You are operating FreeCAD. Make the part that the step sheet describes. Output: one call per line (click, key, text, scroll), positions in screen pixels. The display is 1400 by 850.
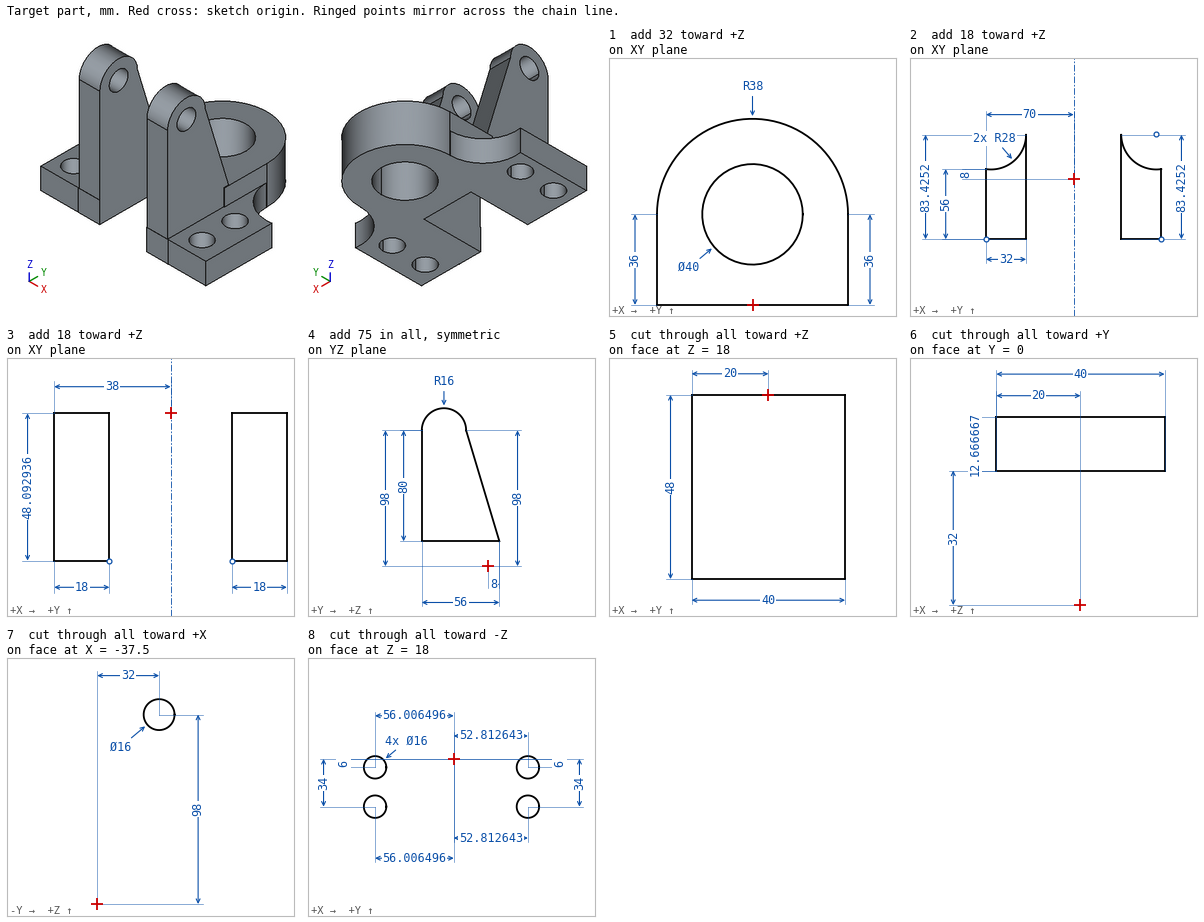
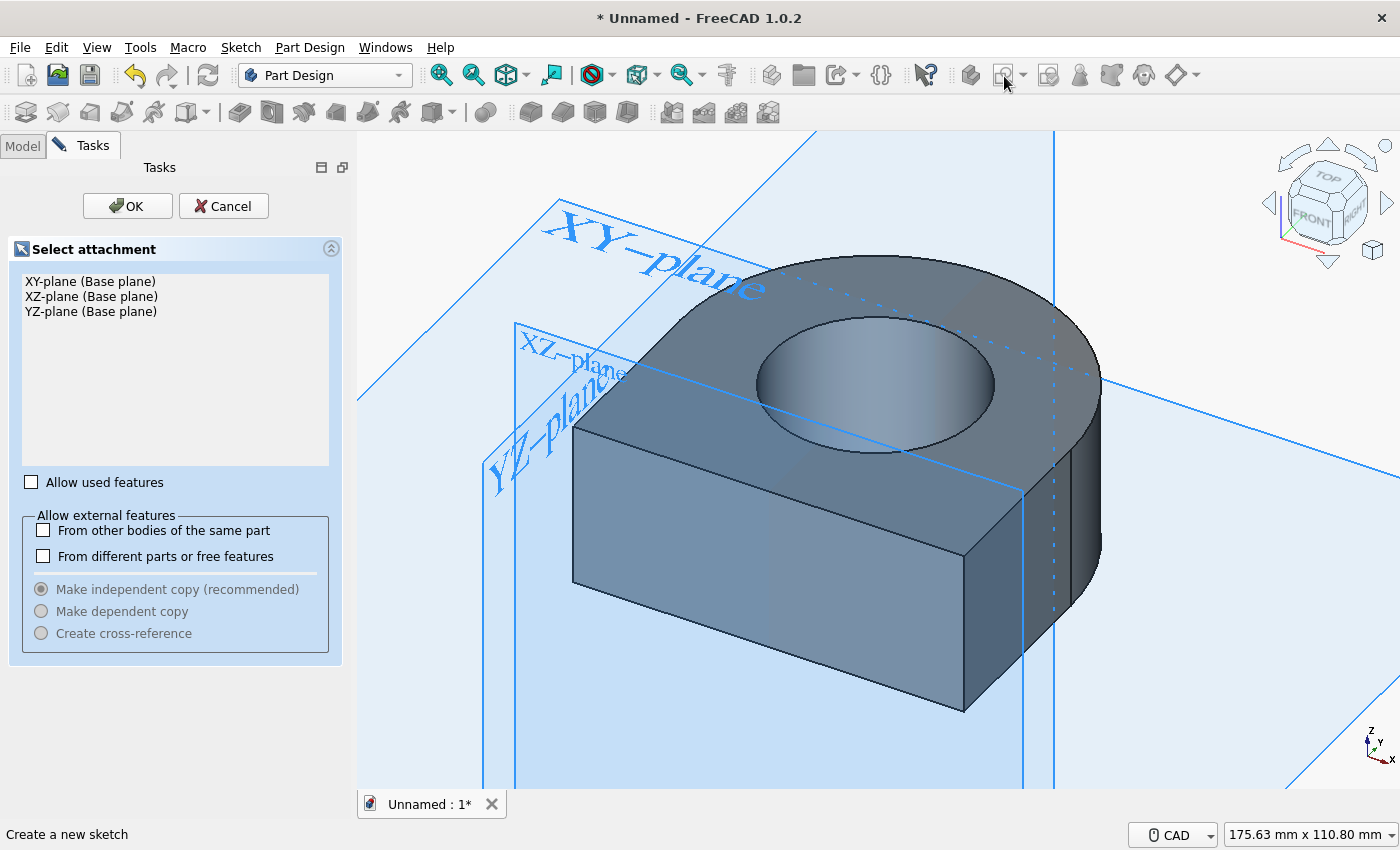
click(82, 282)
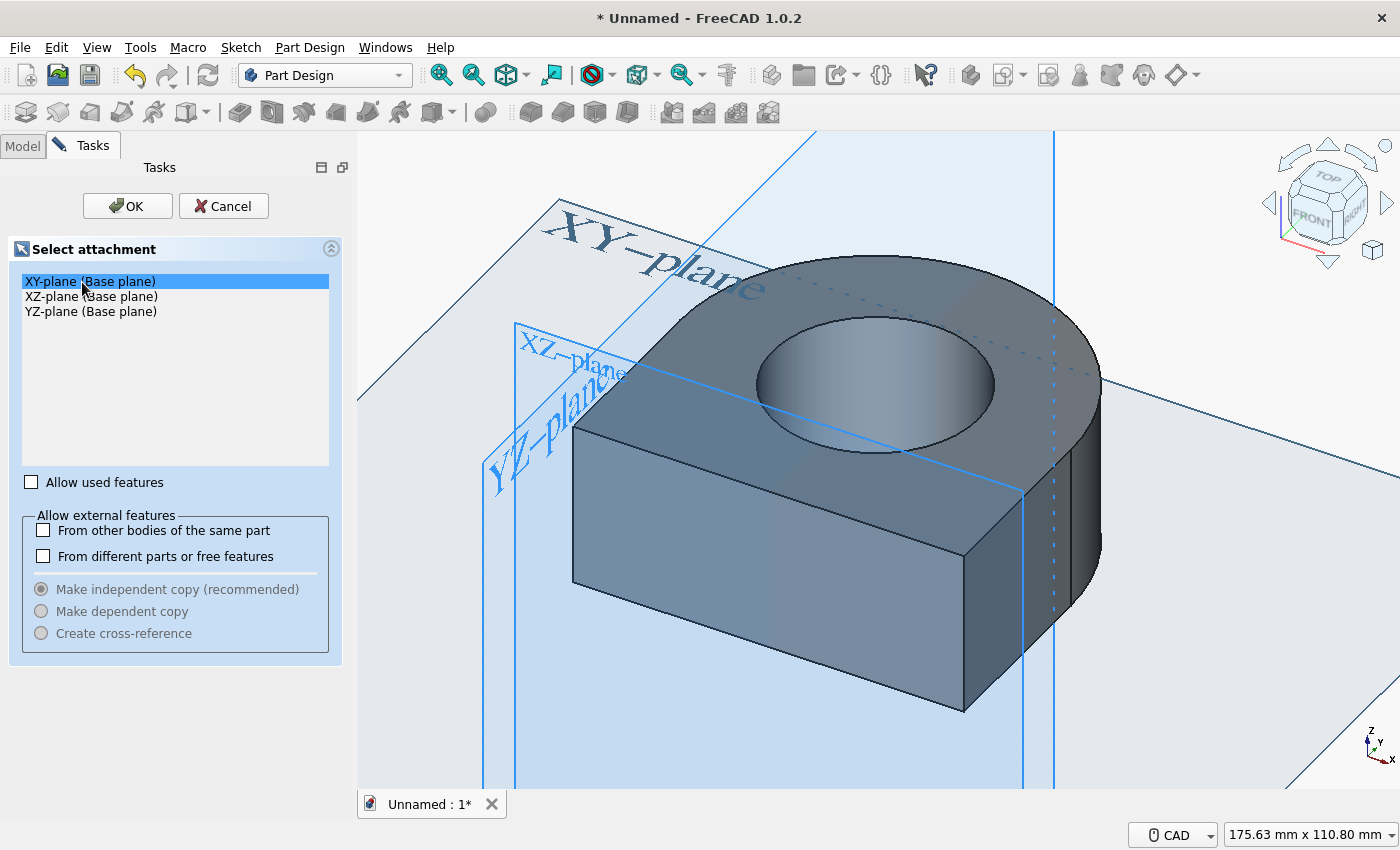
click(128, 206)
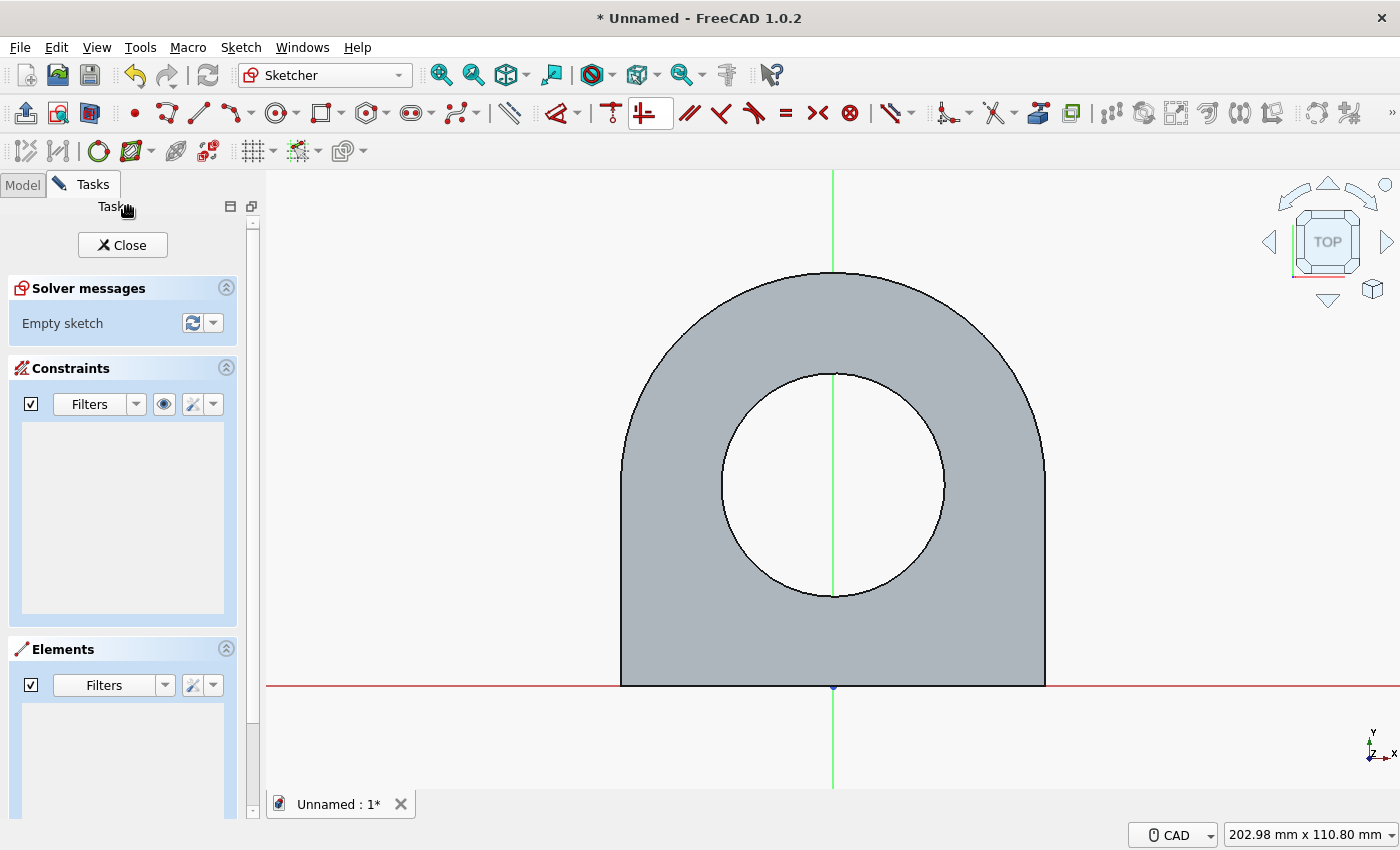
click(90, 114)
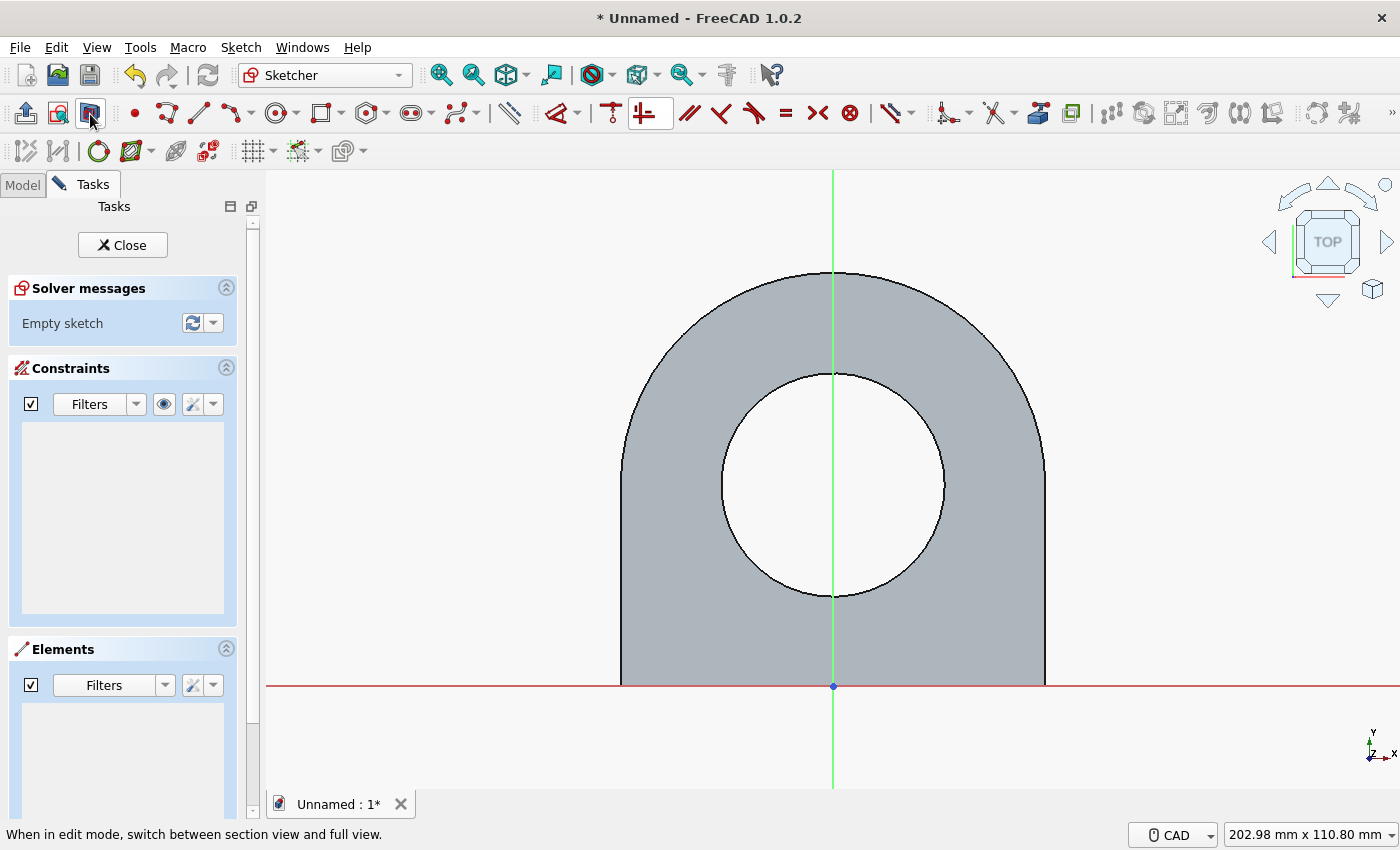
scroll(625, 198, down, 2)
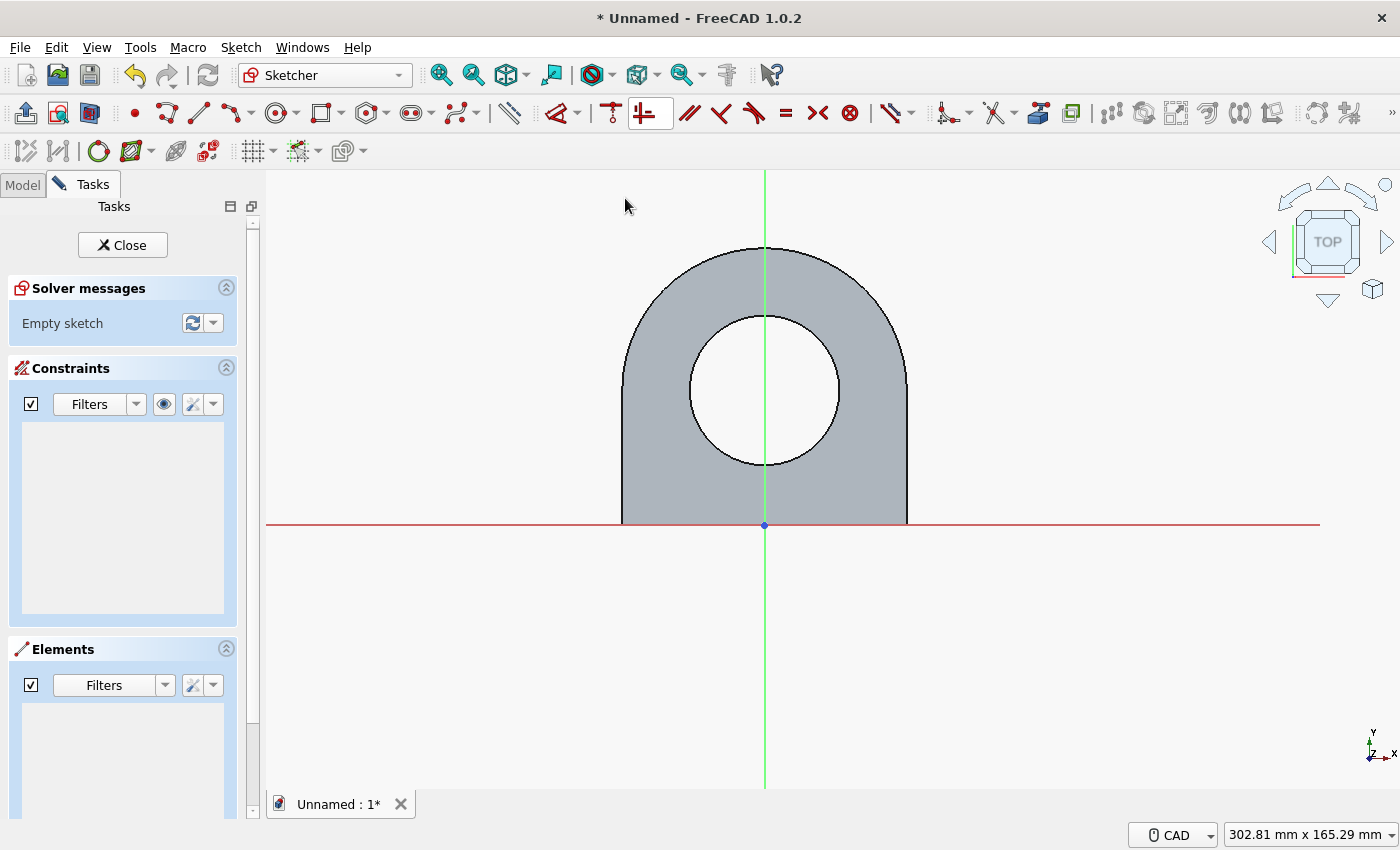
click(168, 114)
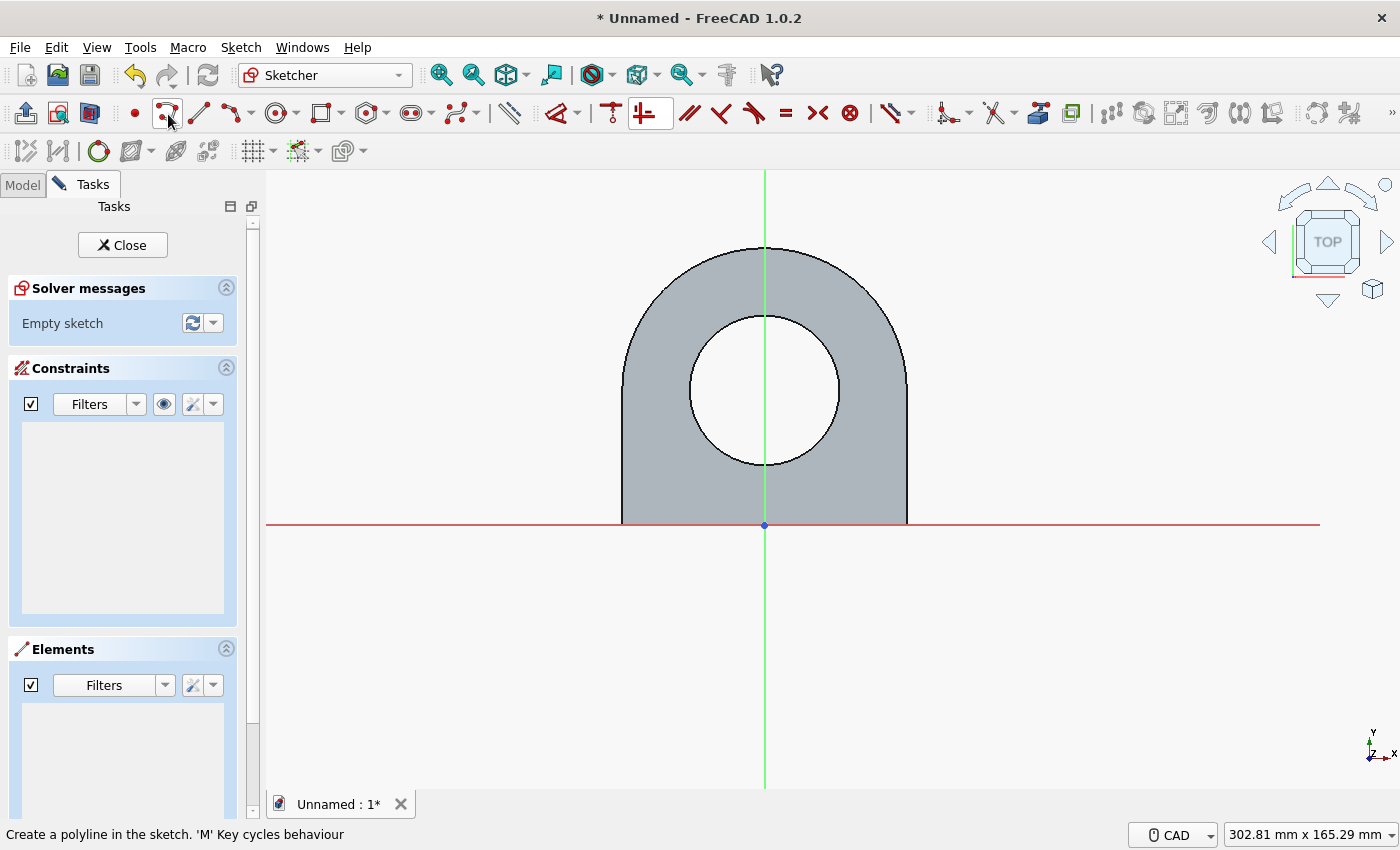
click(502, 495)
click(502, 705)
click(622, 705)
click(622, 393)
right_click(622, 393)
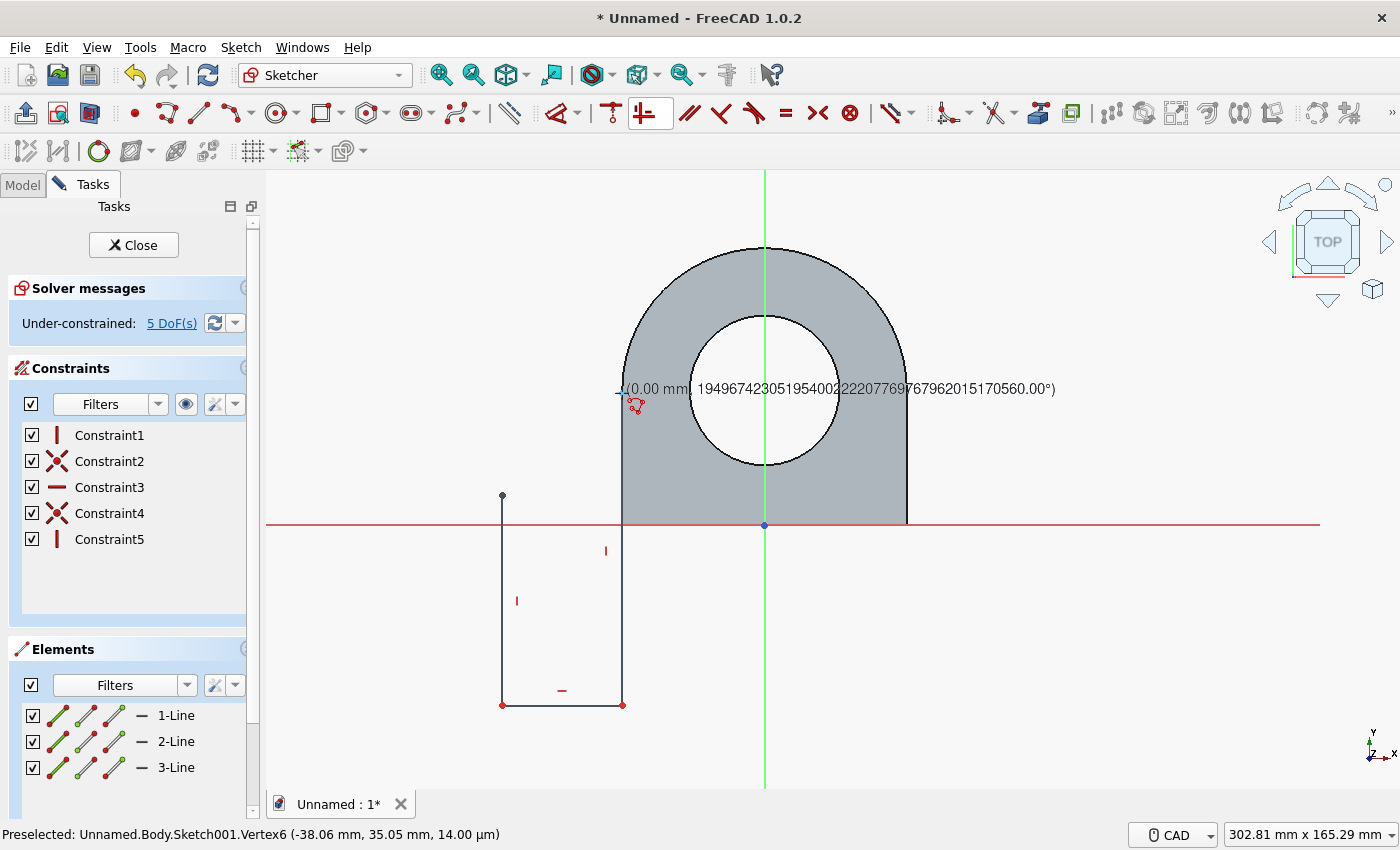
click(232, 114)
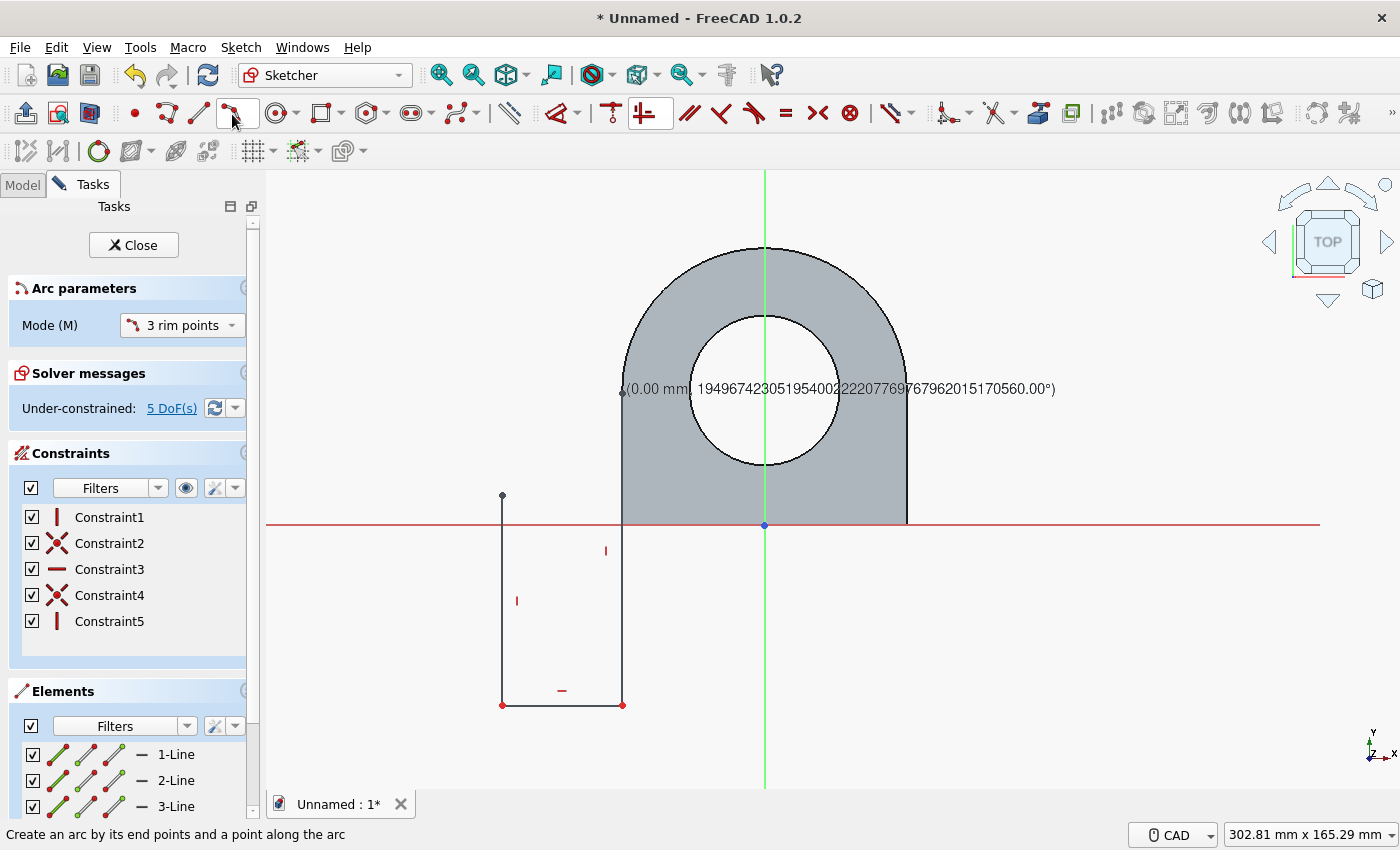
click(622, 394)
click(502, 496)
click(586, 471)